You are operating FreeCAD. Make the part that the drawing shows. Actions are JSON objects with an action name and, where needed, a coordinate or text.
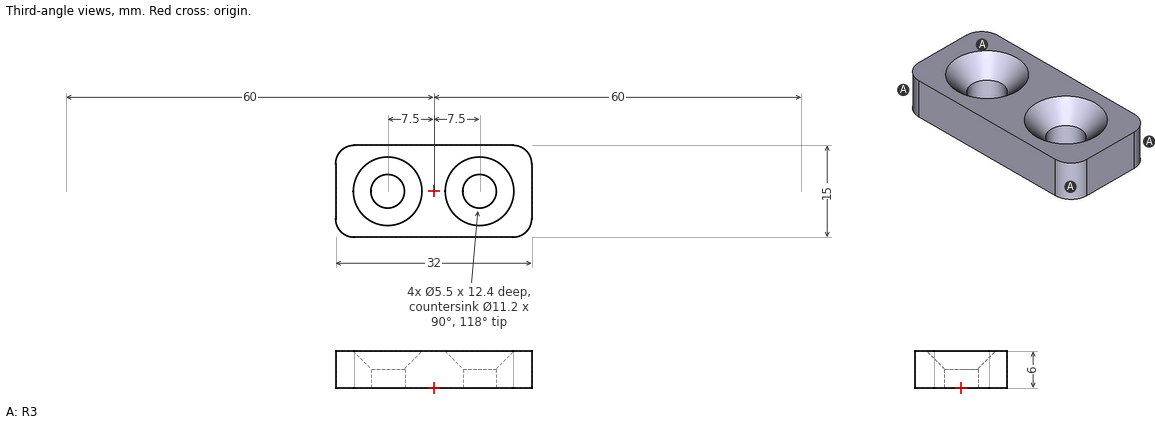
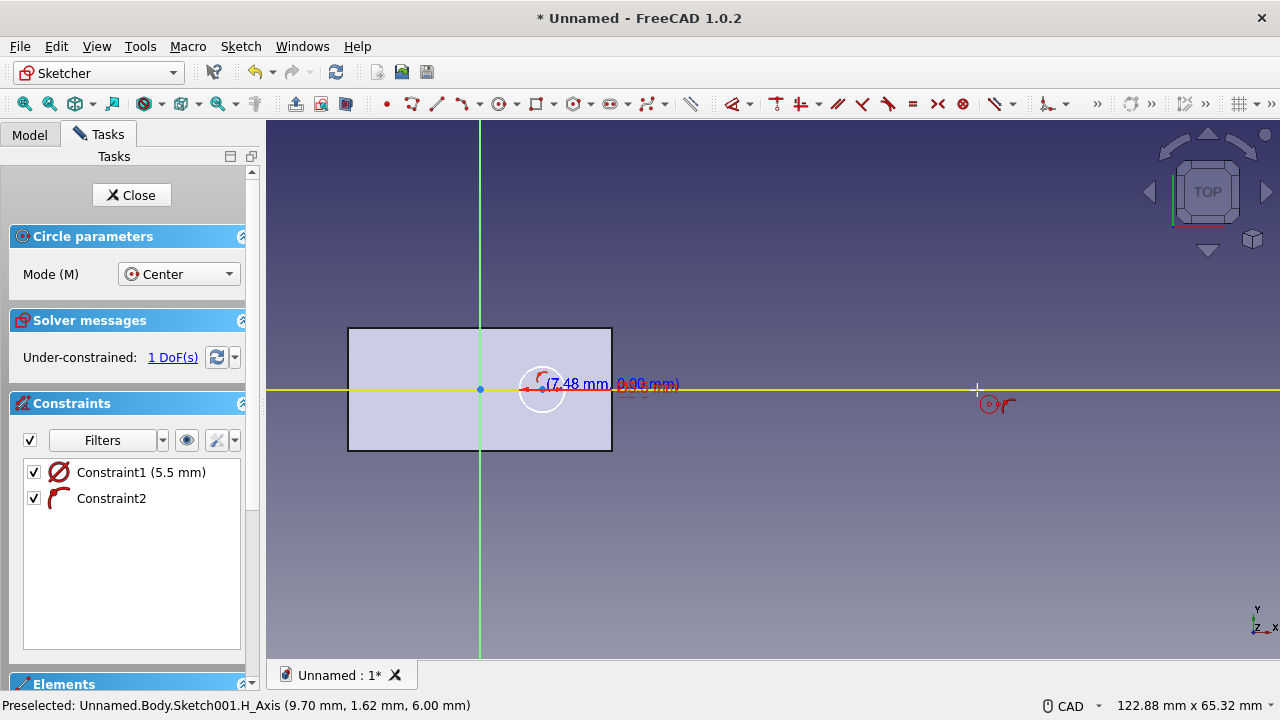
{"action": "left_click", "coordinate": [976, 390]}
{"action": "mouse_move", "coordinate": [992, 373]}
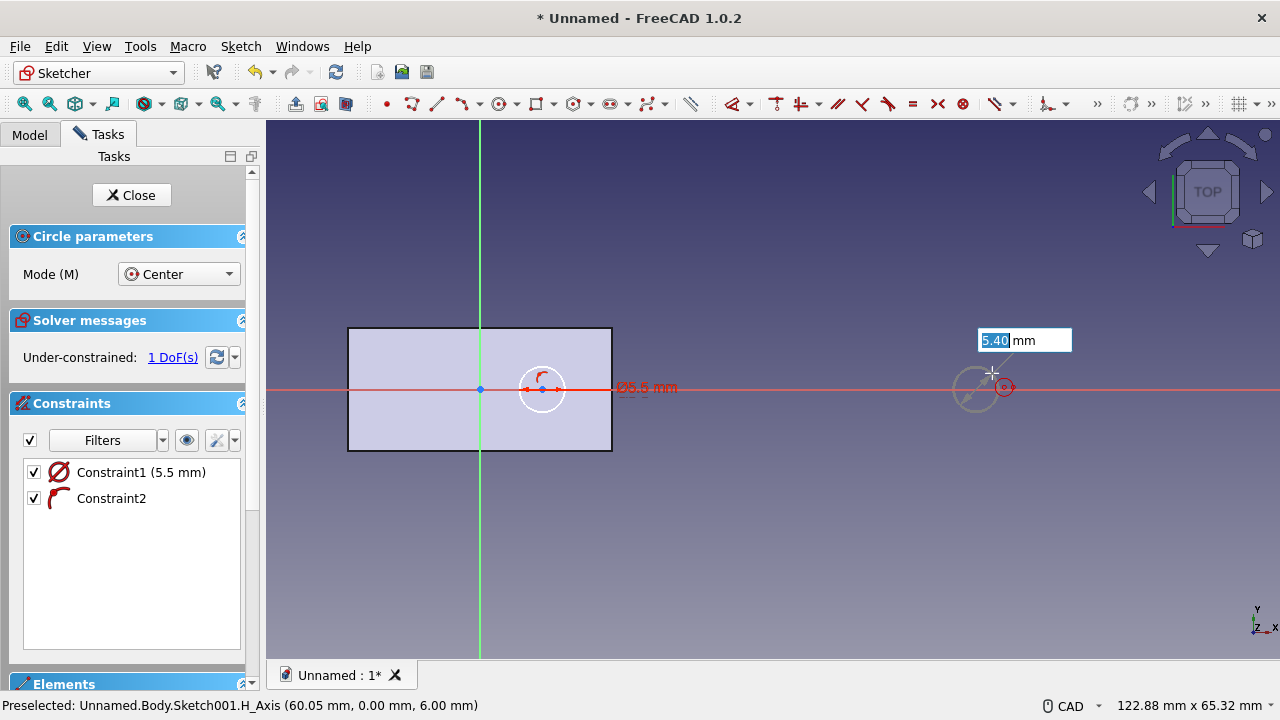
{"action": "type", "text": "5.5"}
{"action": "key", "text": "Return"}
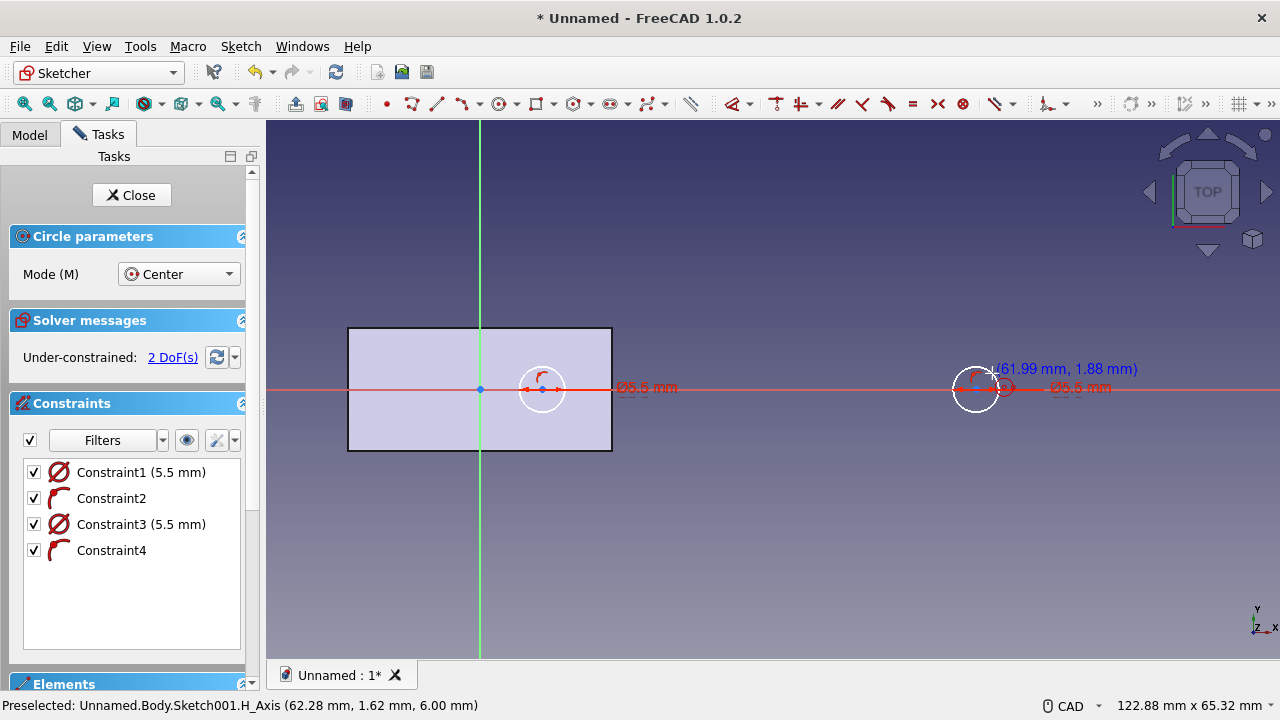
{"action": "scroll", "coordinate": [977, 389], "scroll_direction": "down", "scroll_amount": 3}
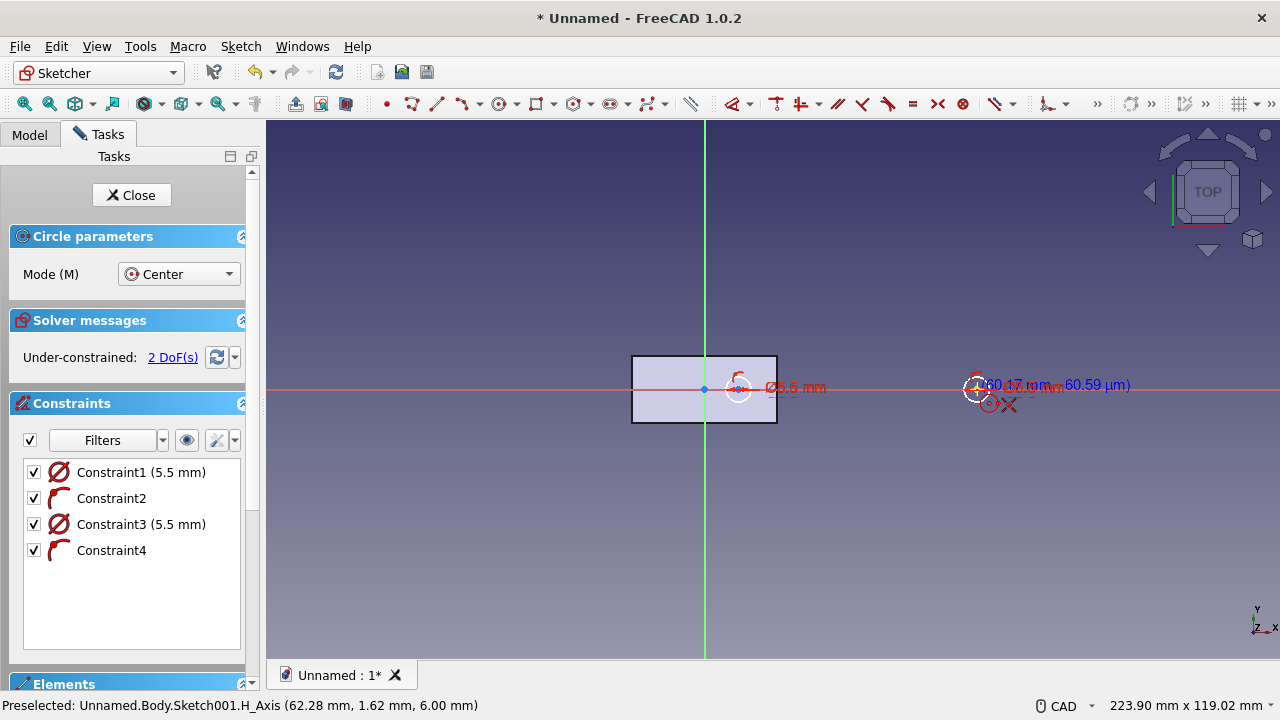
{"action": "scroll", "coordinate": [433, 390], "scroll_direction": "up", "scroll_amount": 3}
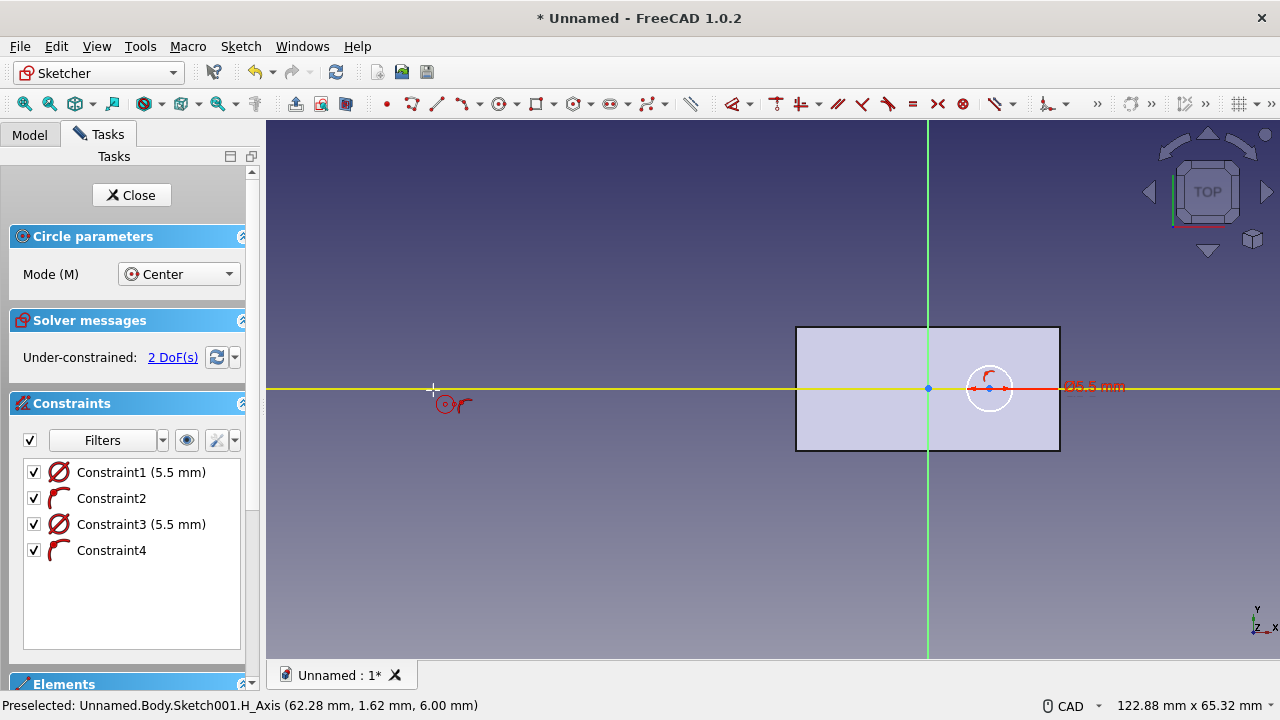
{"action": "left_click", "coordinate": [433, 389]}
{"action": "mouse_move", "coordinate": [449, 373]}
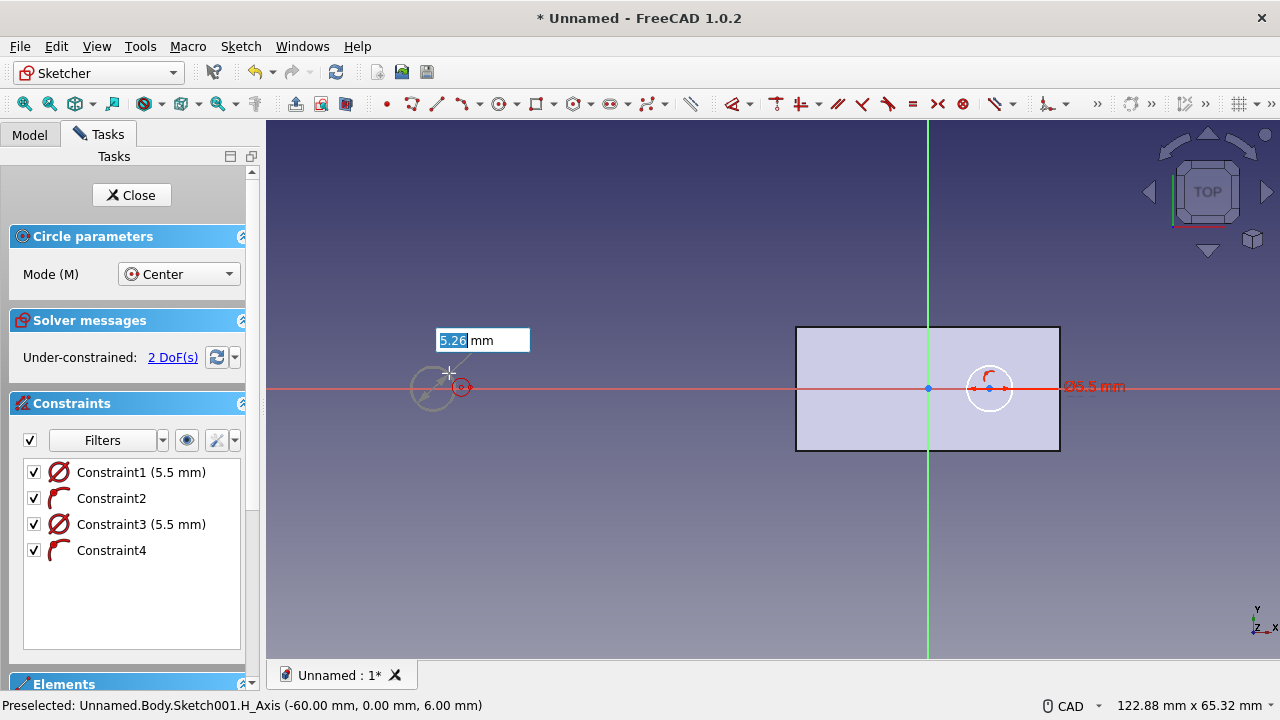
{"action": "type", "text": "5.5"}
{"action": "key", "text": "Return"}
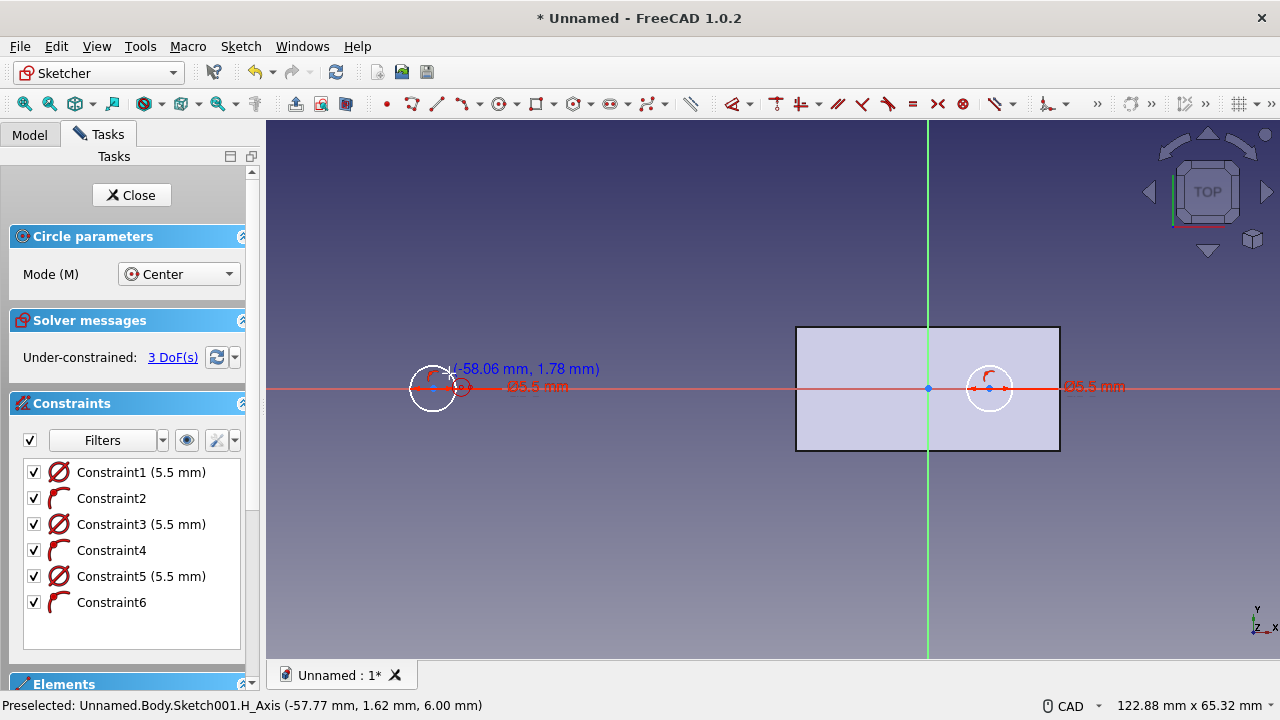
{"action": "left_click", "coordinate": [866, 389]}
{"action": "mouse_move", "coordinate": [882, 373]}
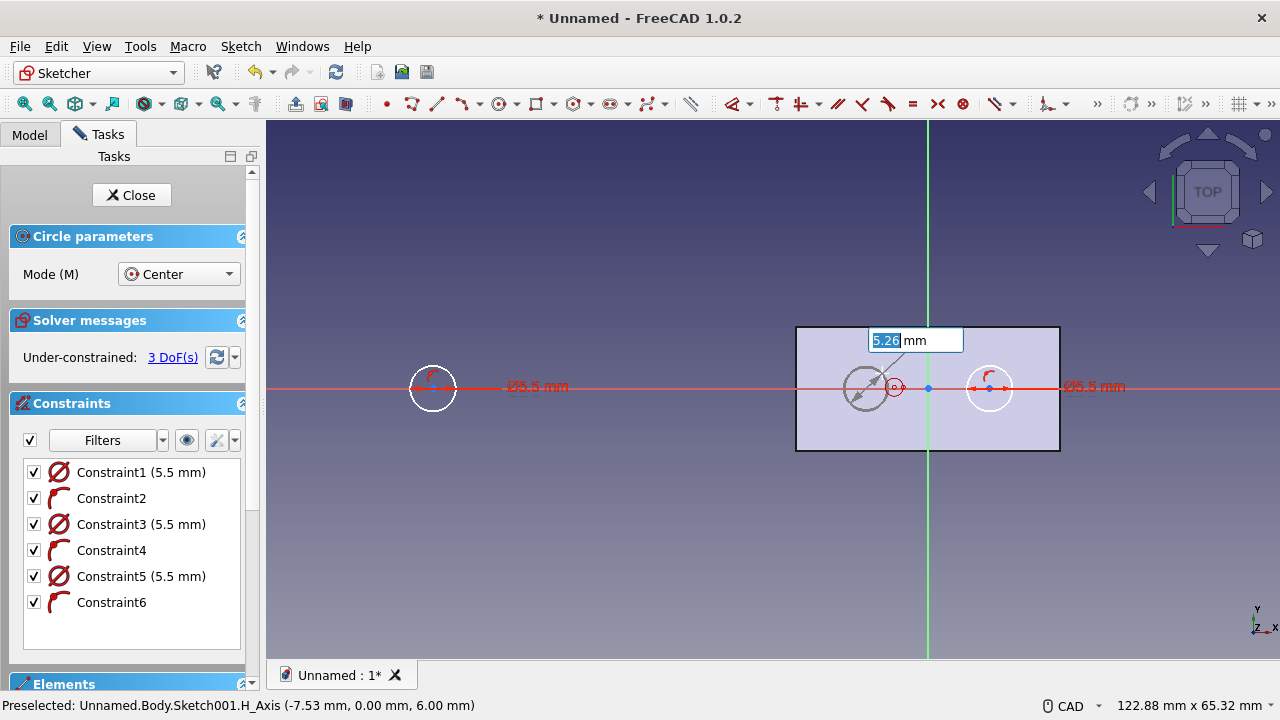
{"action": "type", "text": "5.5"}
{"action": "key", "text": "Return"}
{"action": "key", "text": "Escape"}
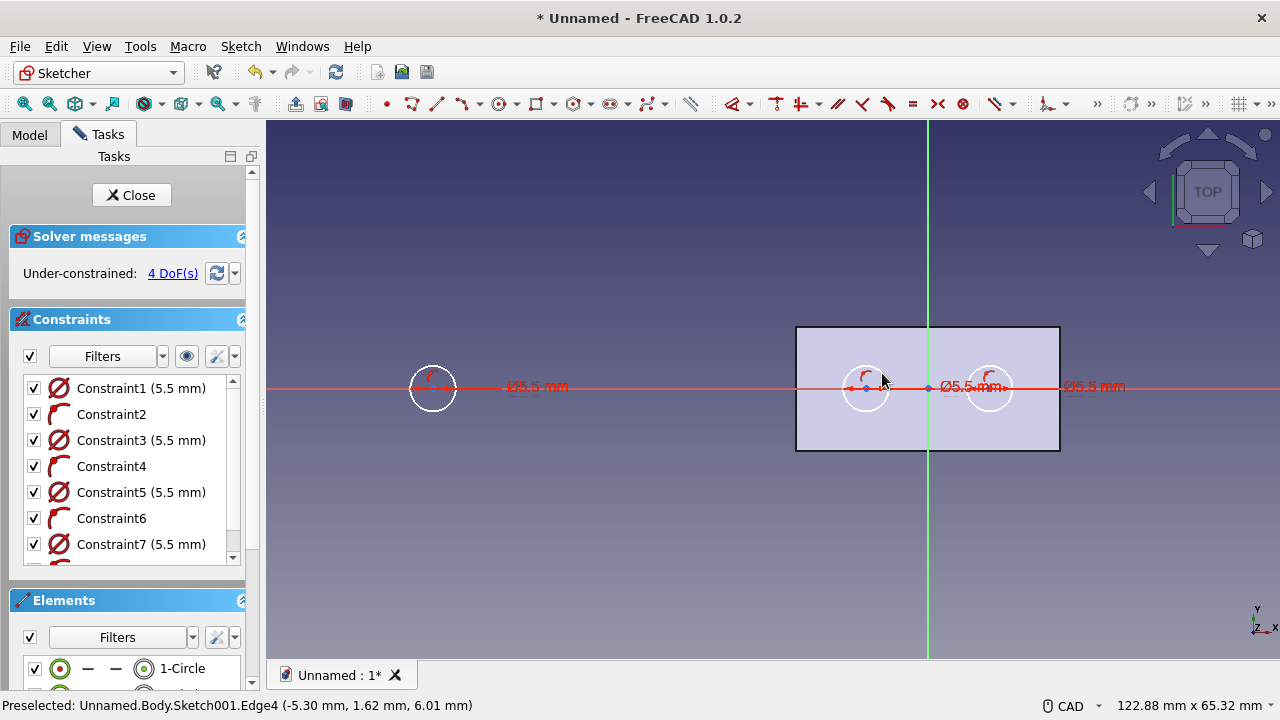
{"action": "left_click", "coordinate": [732, 104]}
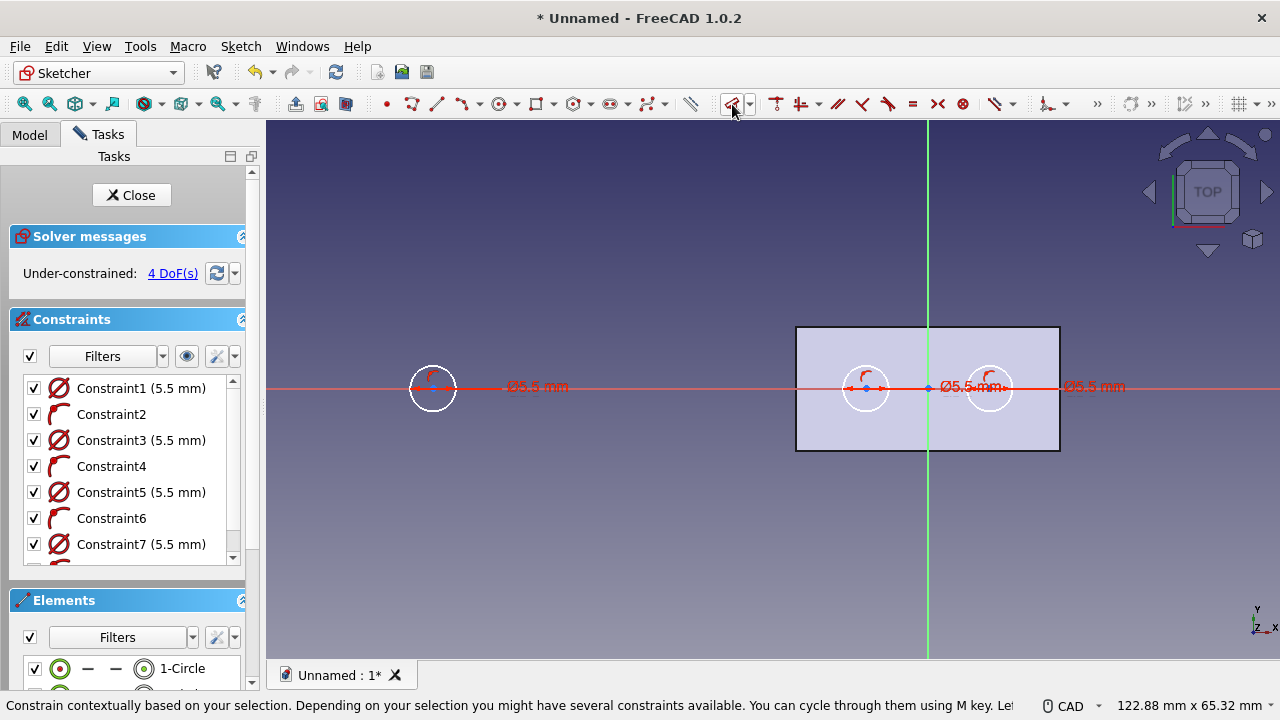
{"action": "scroll", "coordinate": [433, 391], "scroll_direction": "down", "scroll_amount": 3}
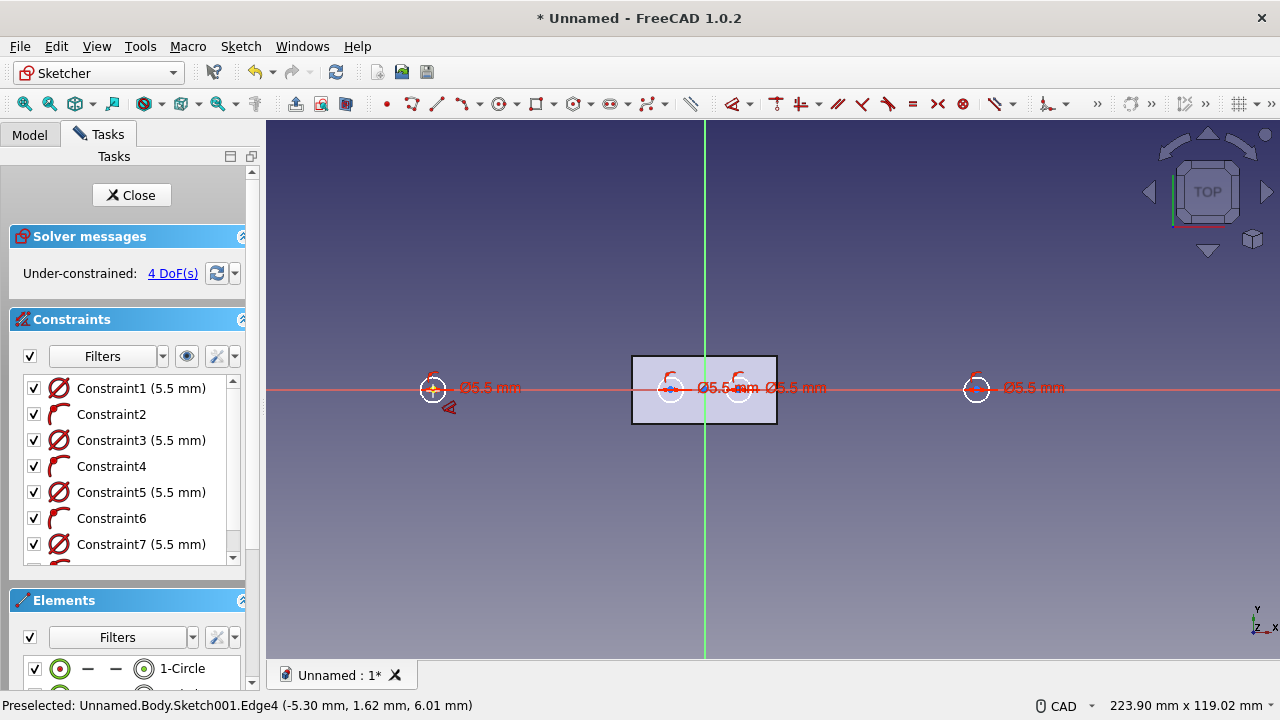
{"action": "left_click", "coordinate": [977, 390]}
{"action": "left_click", "coordinate": [841, 424]}